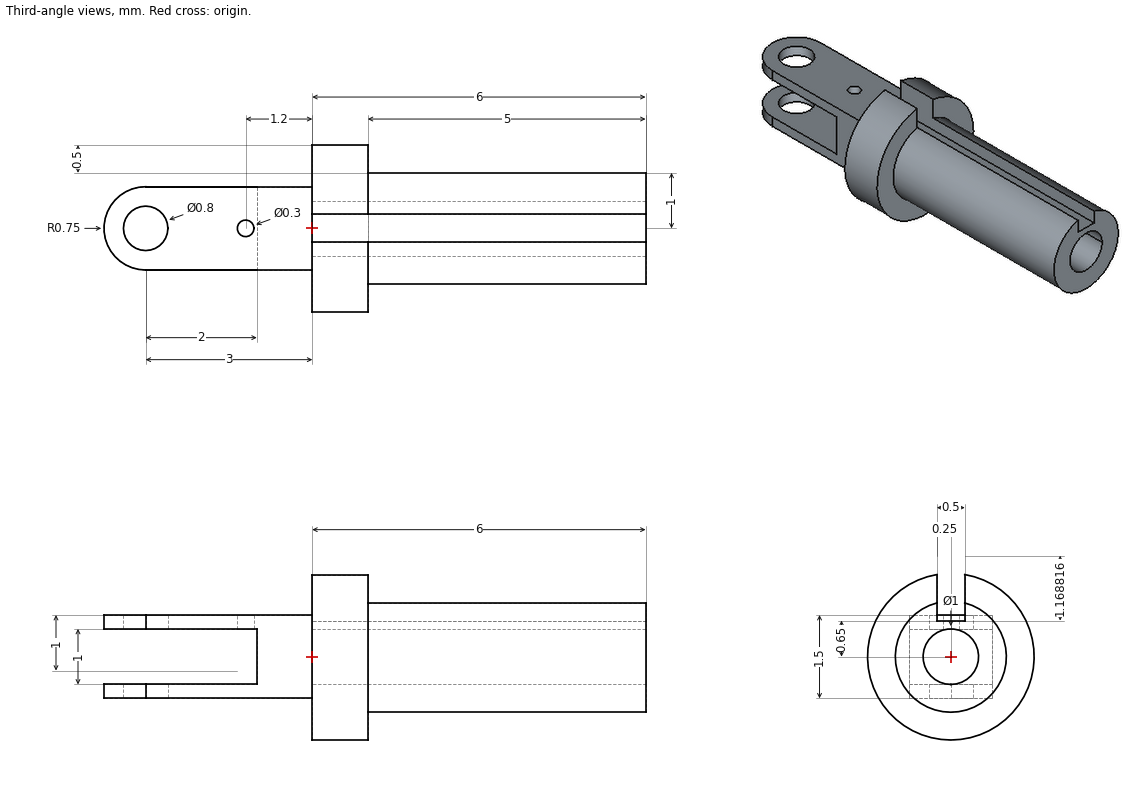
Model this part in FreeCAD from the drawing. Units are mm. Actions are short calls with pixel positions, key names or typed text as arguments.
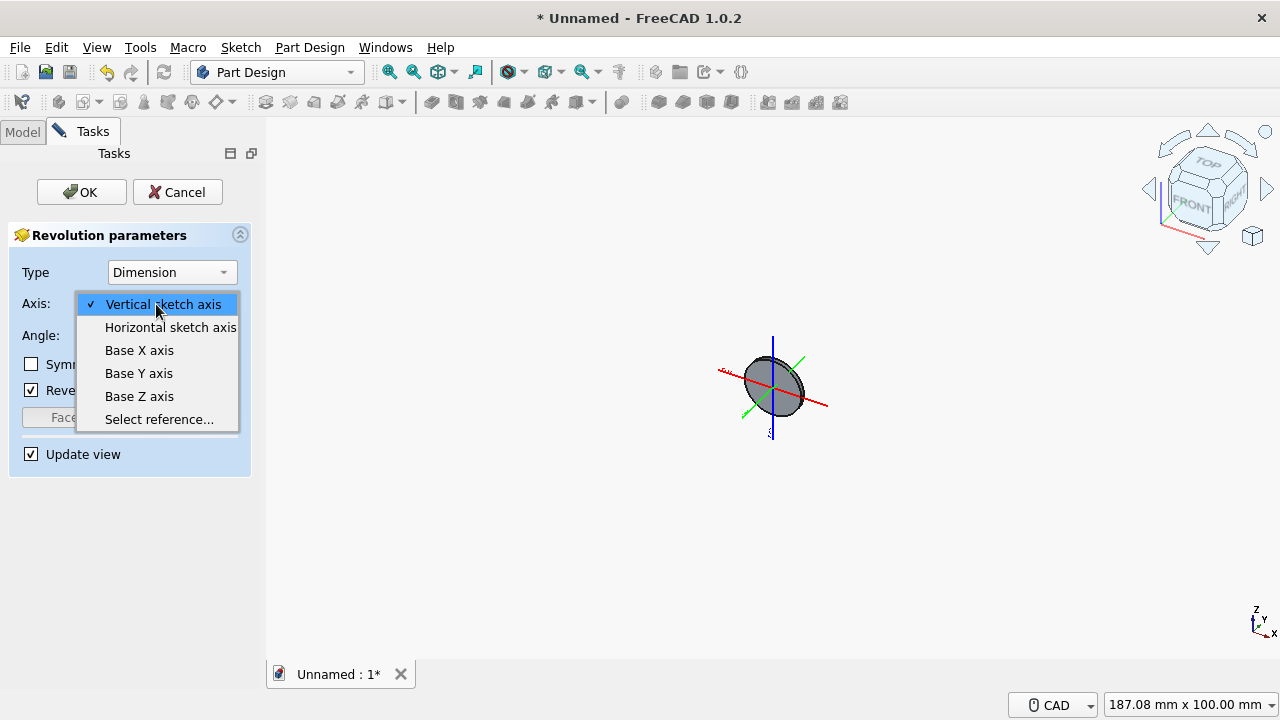
click(156, 328)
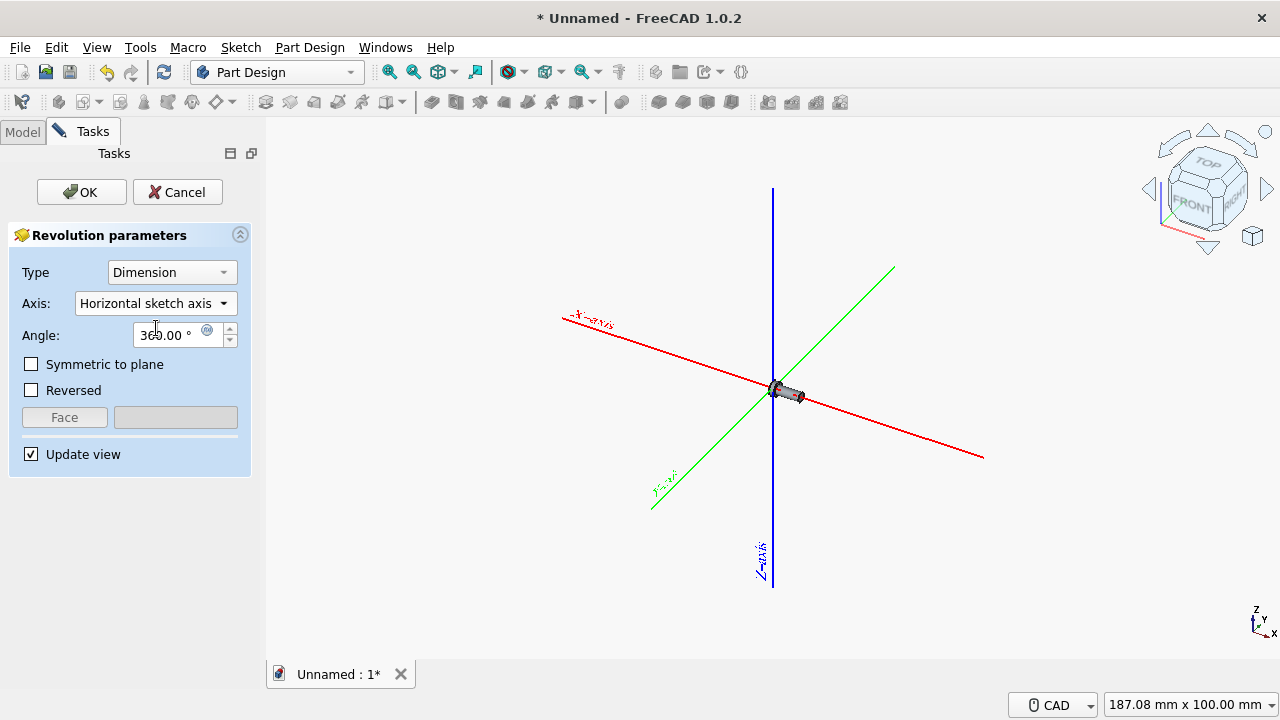
click(82, 192)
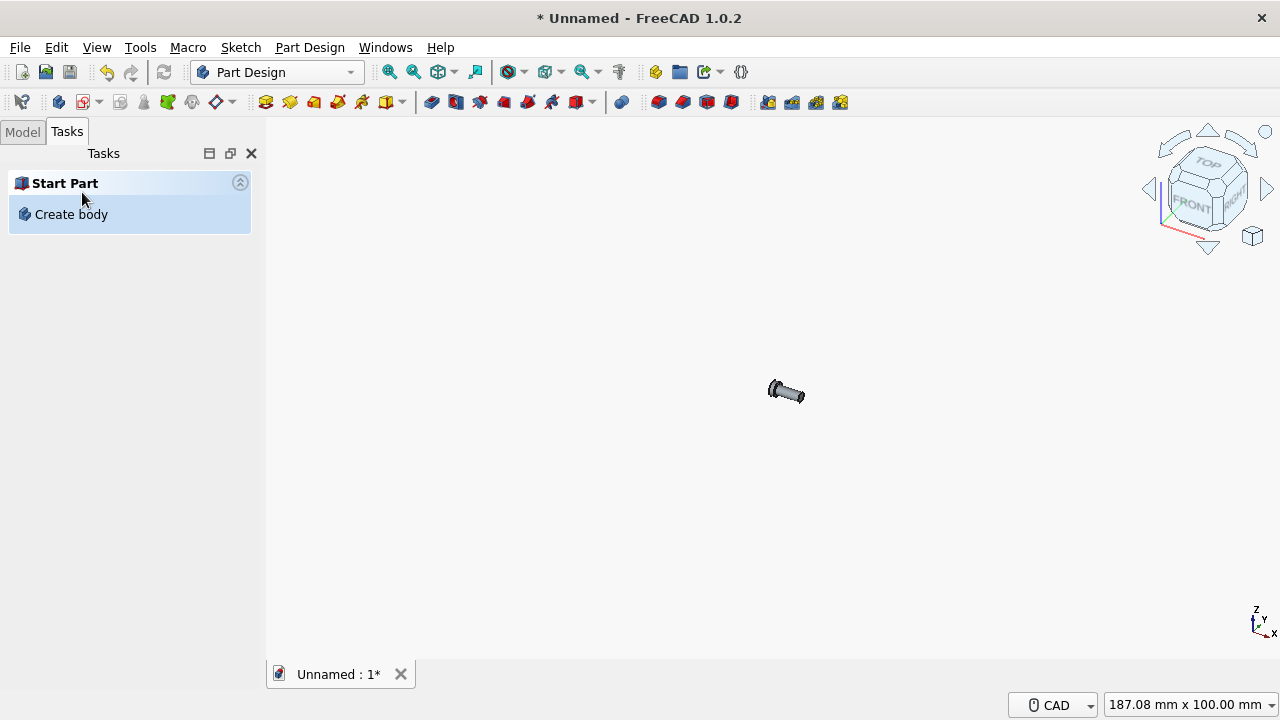
click(390, 72)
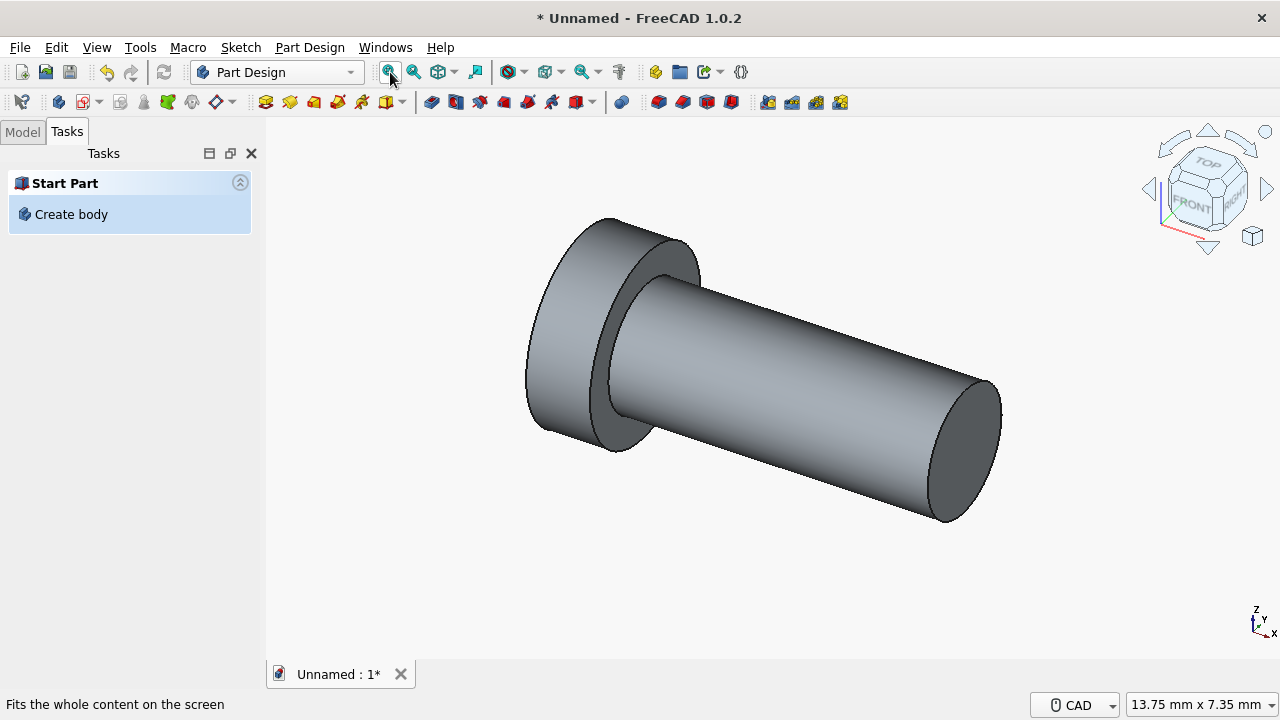
click(84, 102)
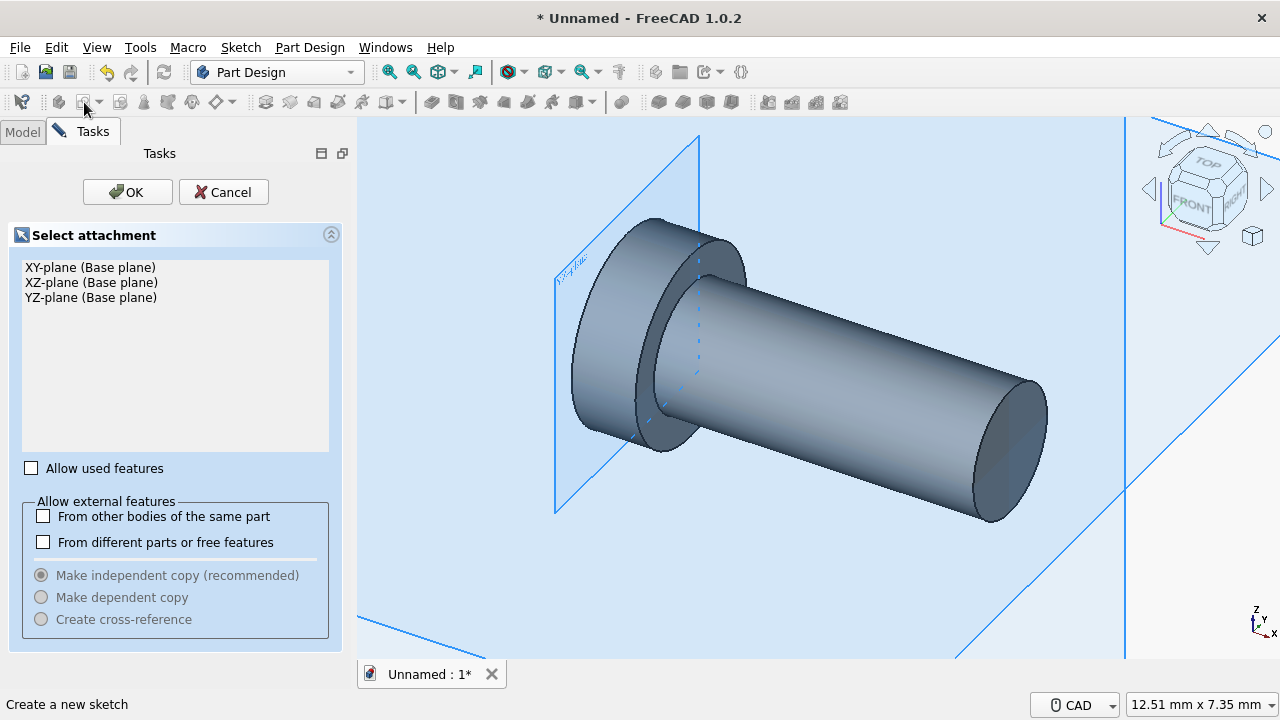
click(82, 268)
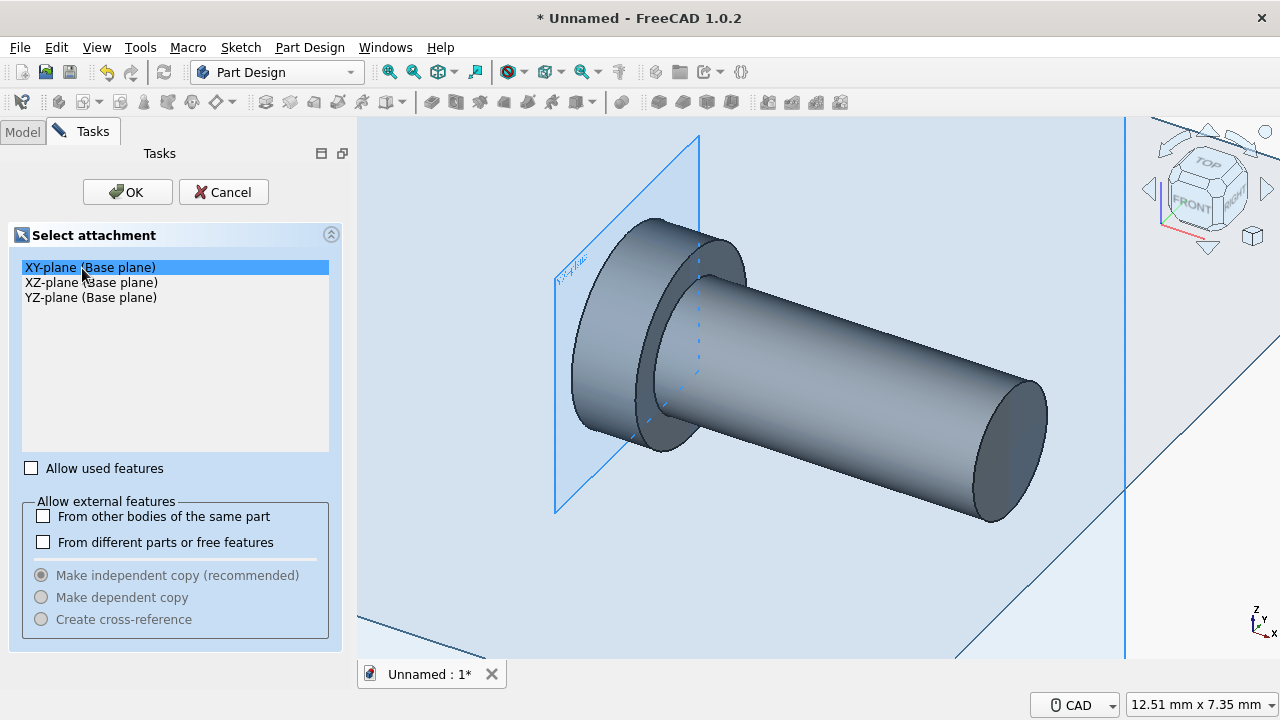
click(128, 192)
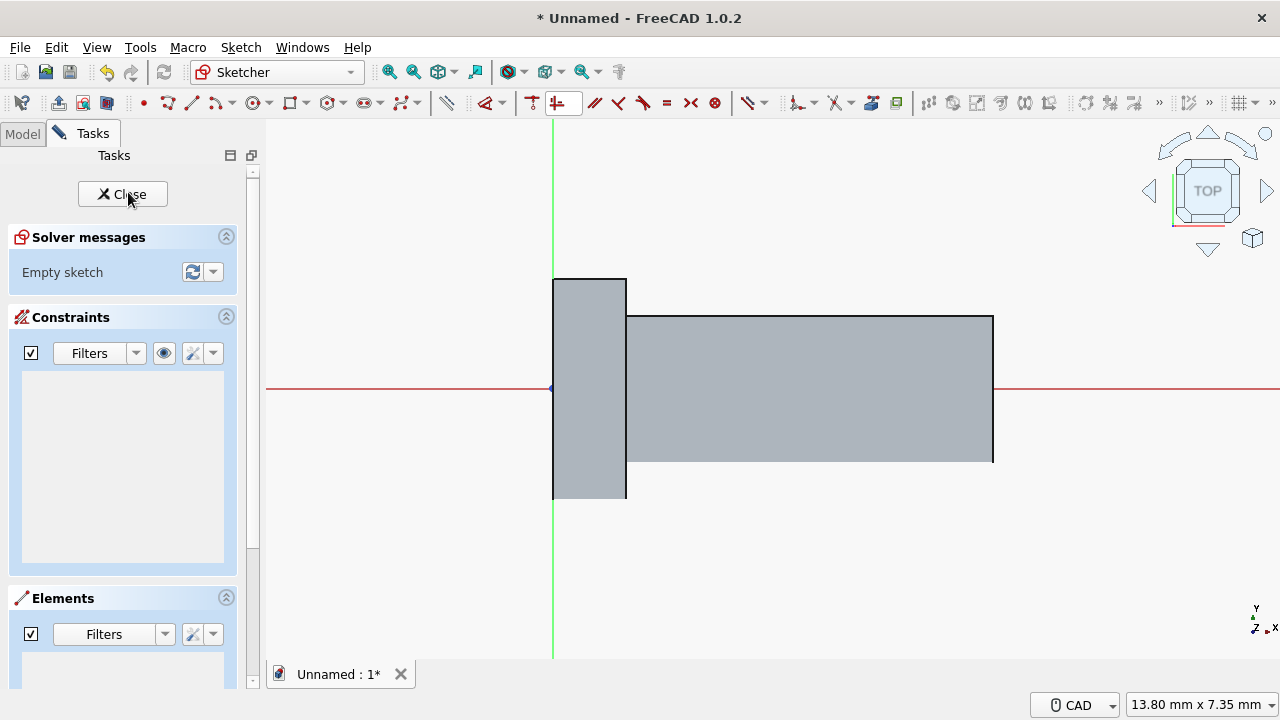
click(108, 104)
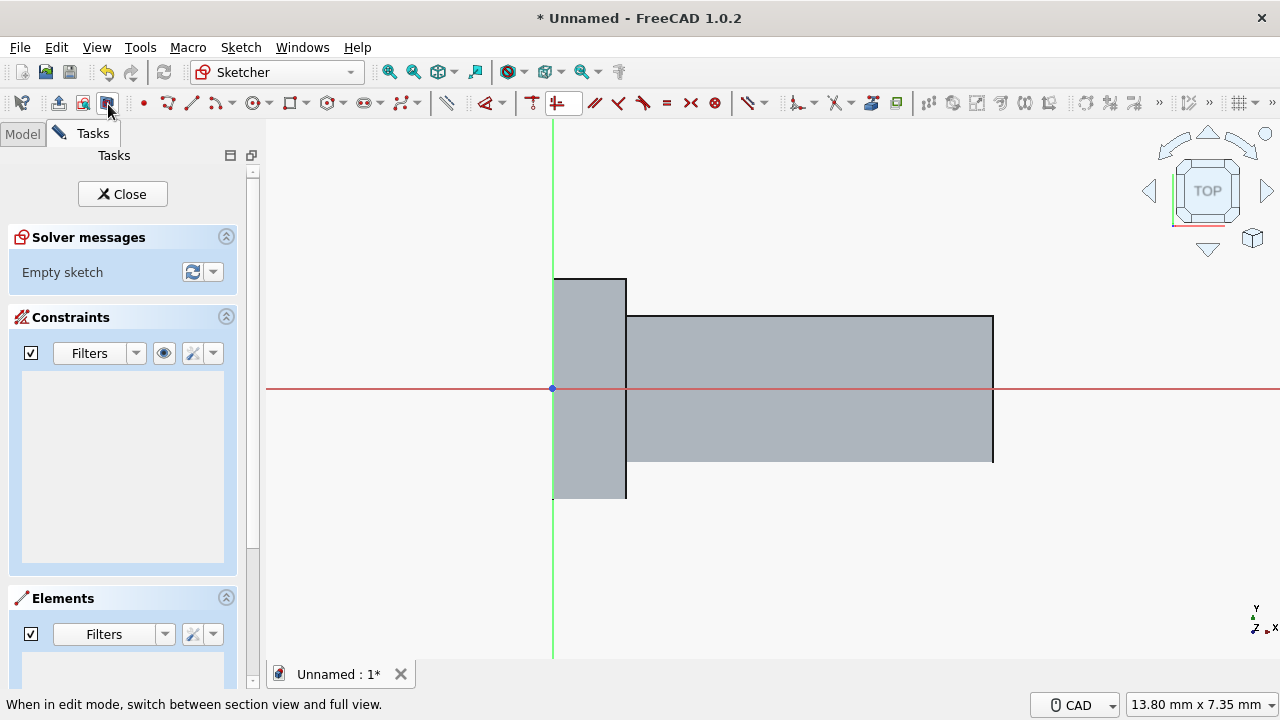
scroll(704, 389, down, 5)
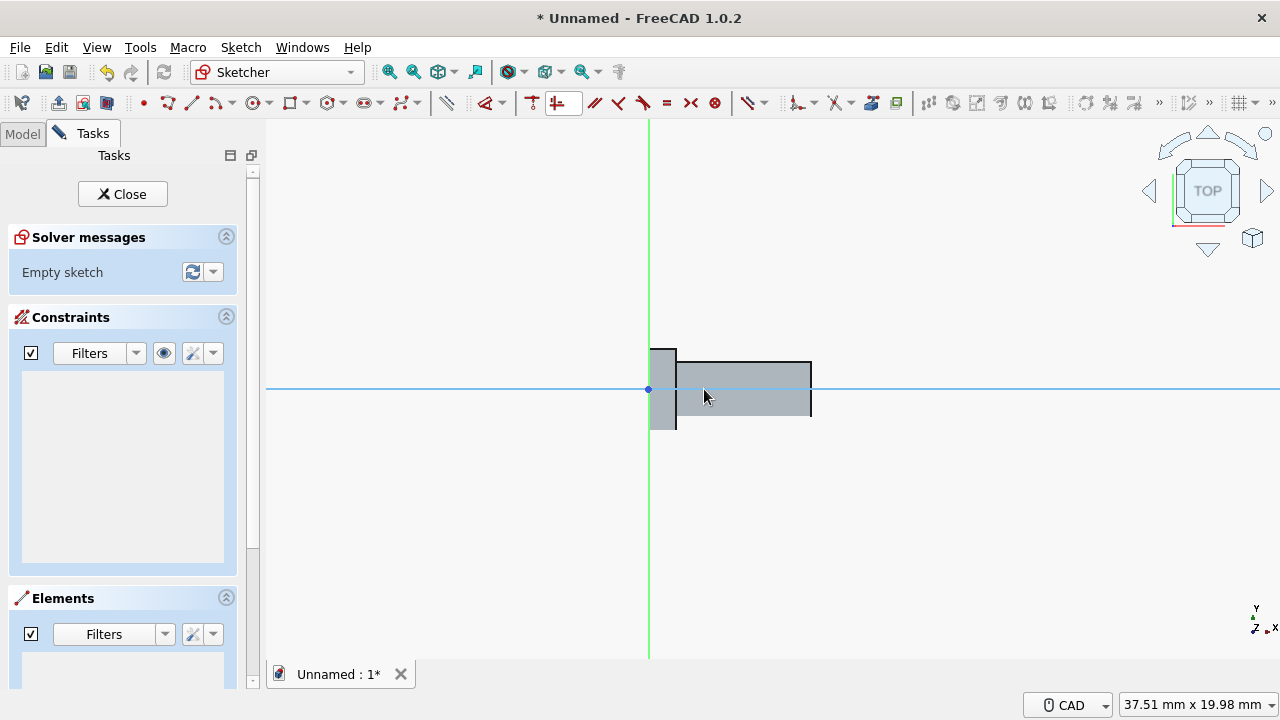
scroll(577, 389, up, 9)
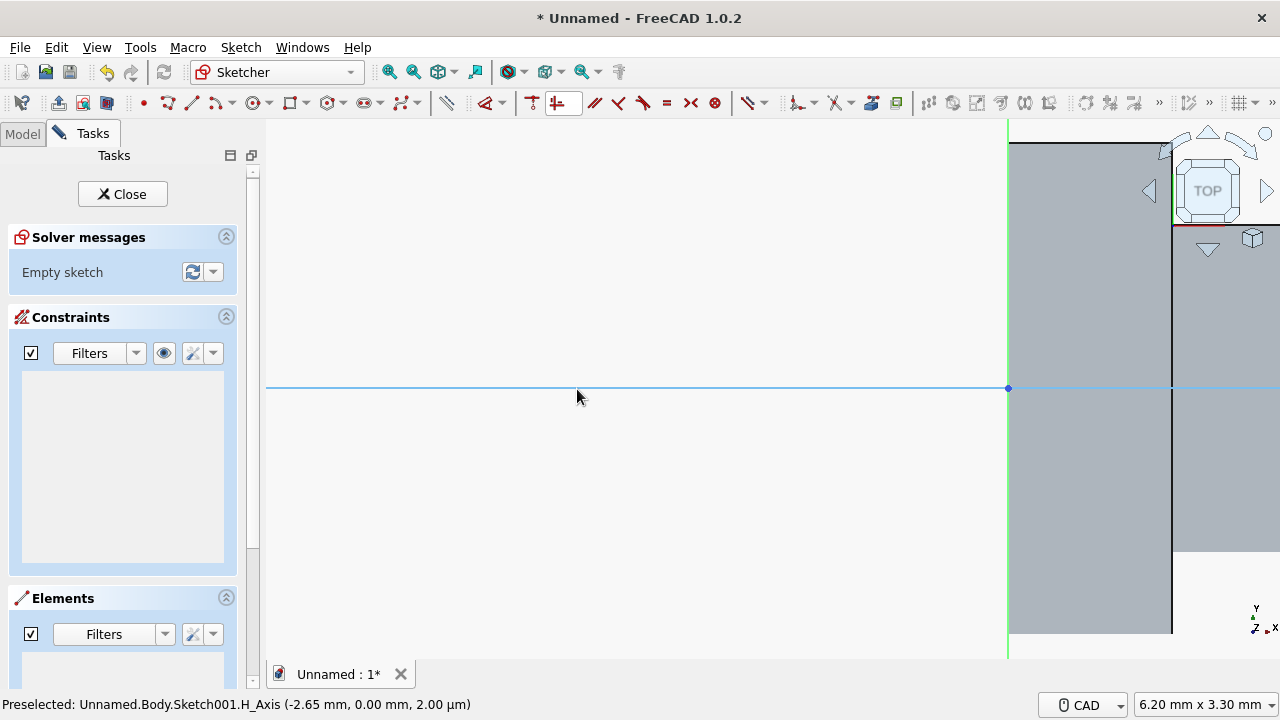
click(168, 104)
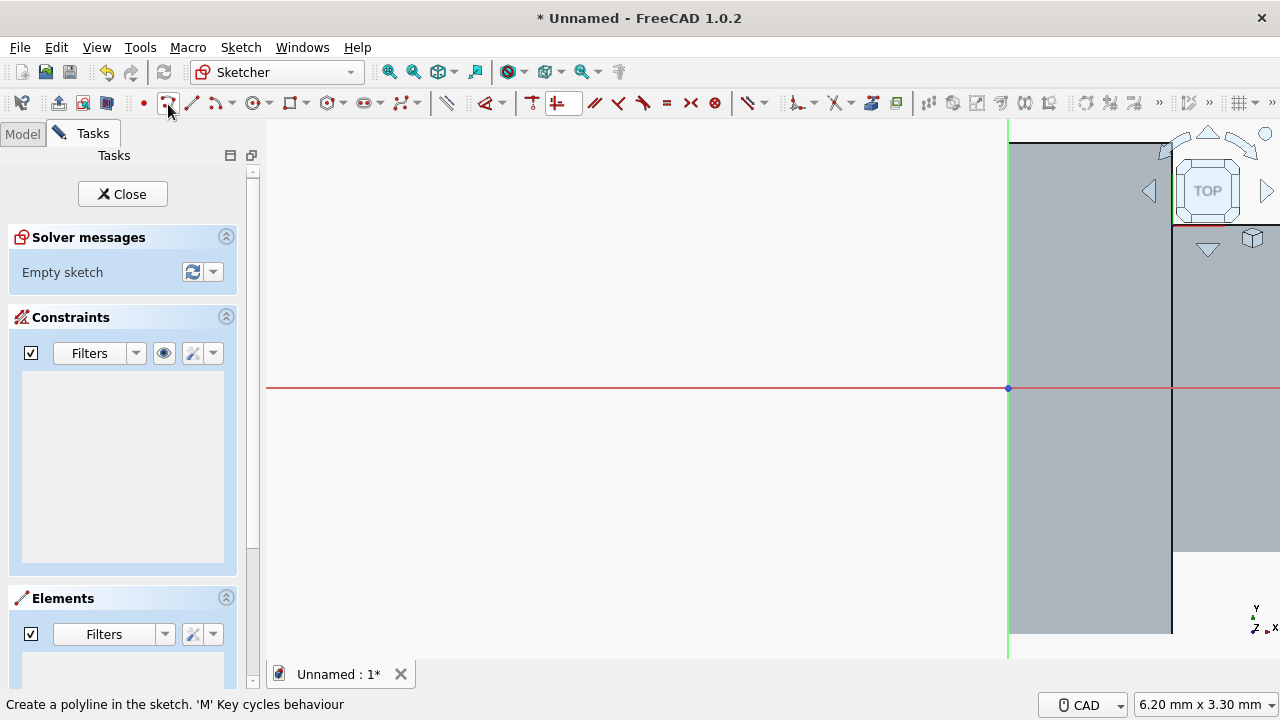
click(518, 511)
click(1008, 511)
click(999, 266)
click(518, 266)
right_click(518, 266)